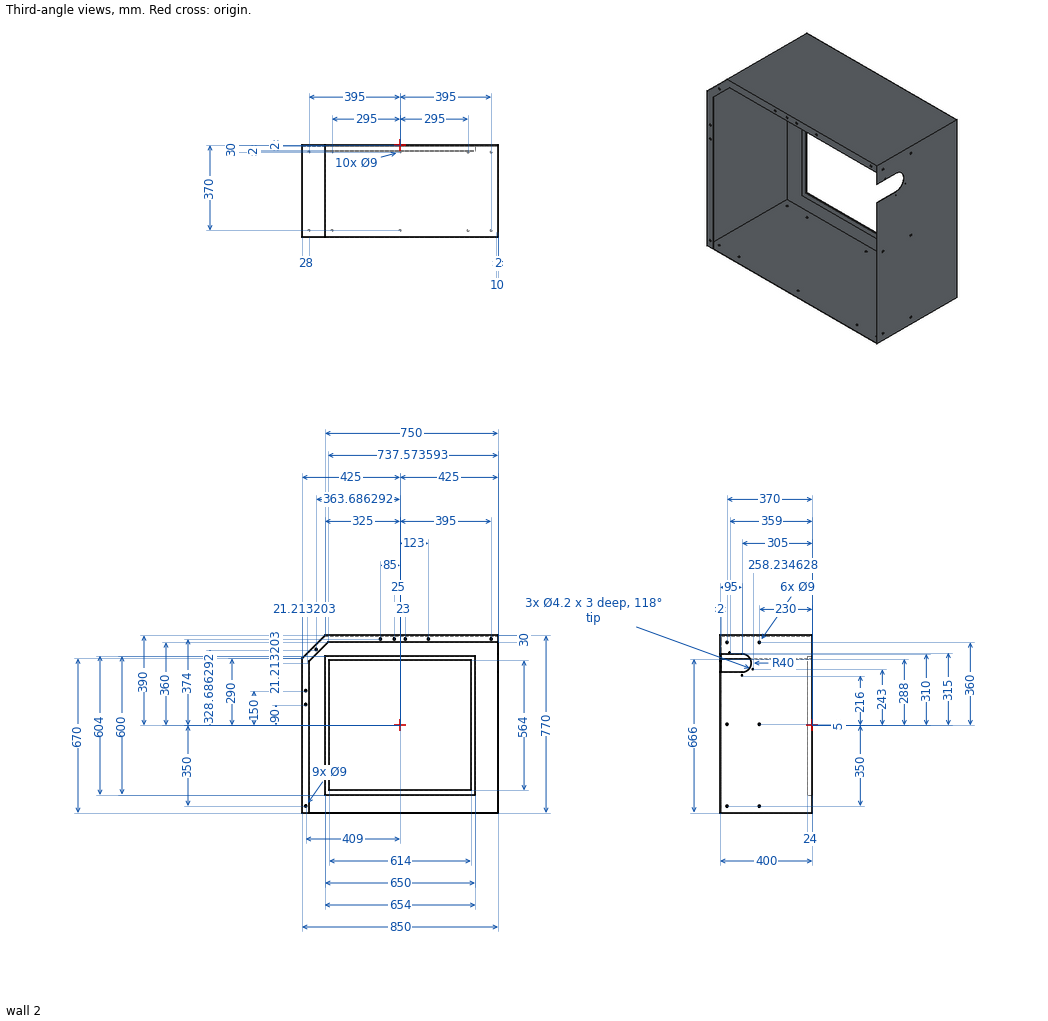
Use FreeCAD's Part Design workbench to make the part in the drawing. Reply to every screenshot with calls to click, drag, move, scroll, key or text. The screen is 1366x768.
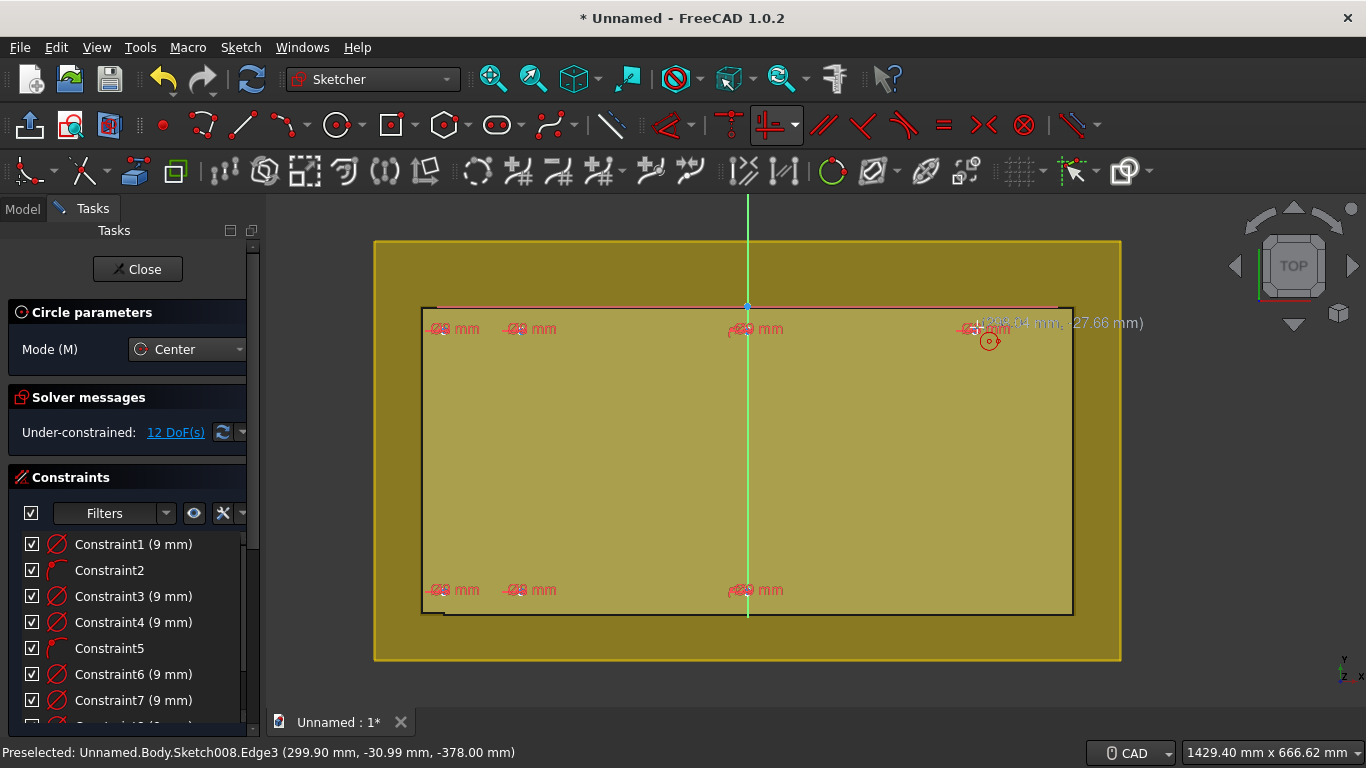
scroll(975, 591, up, 10)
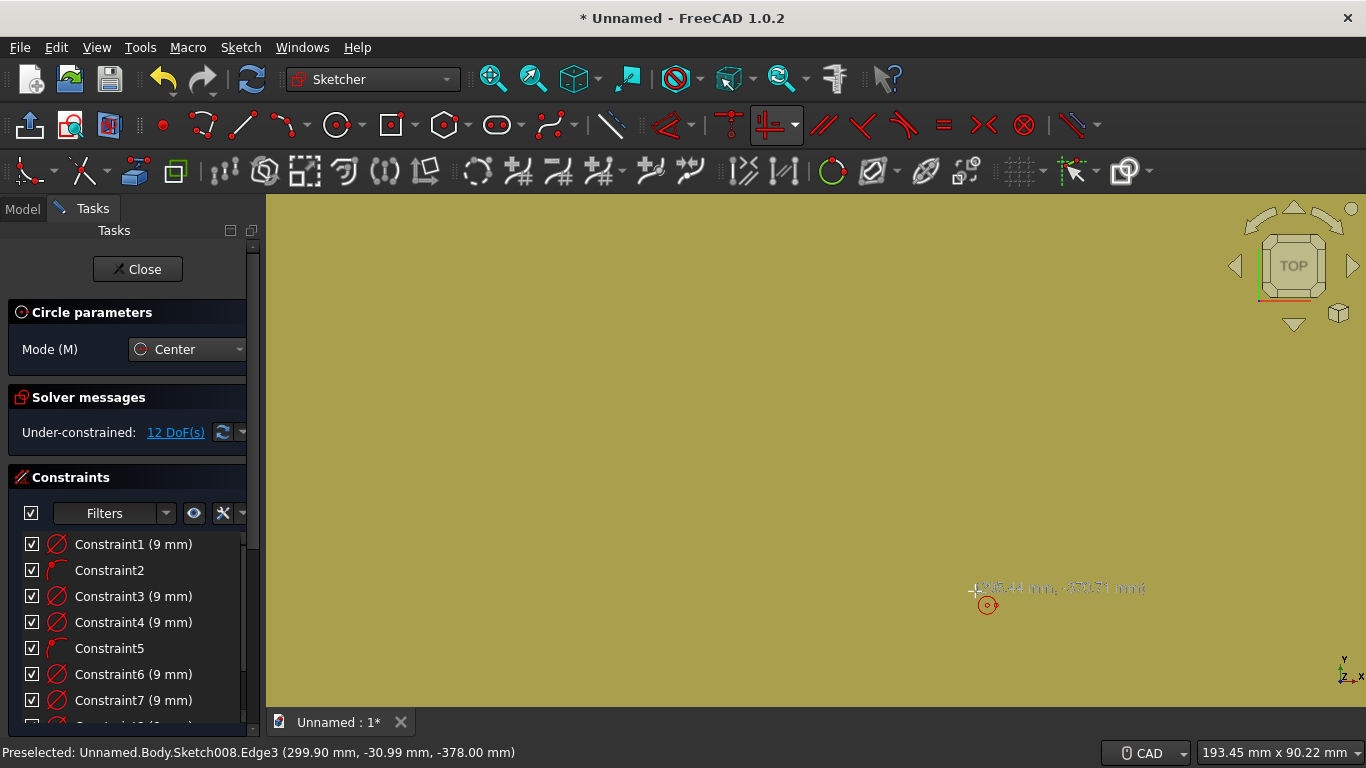
scroll(975, 591, down, 10)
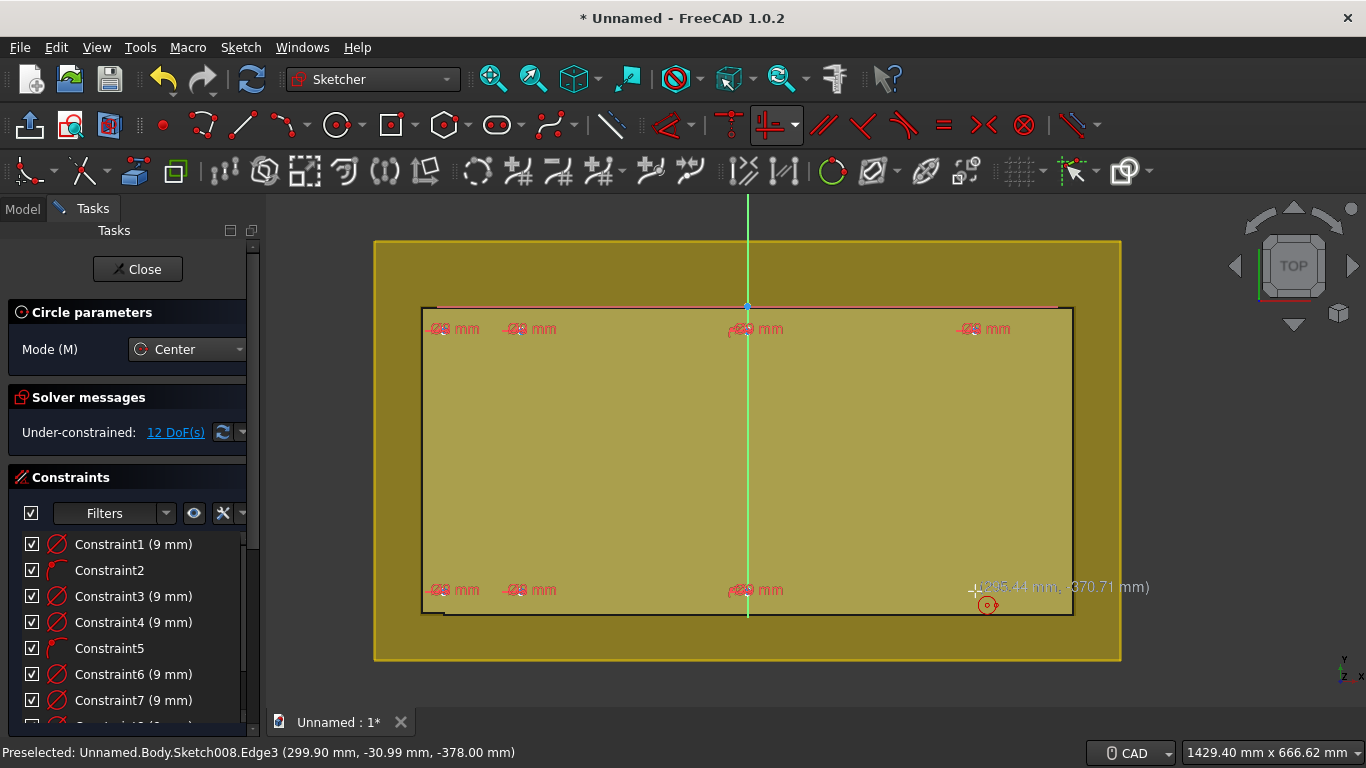
click(975, 591)
move(977, 589)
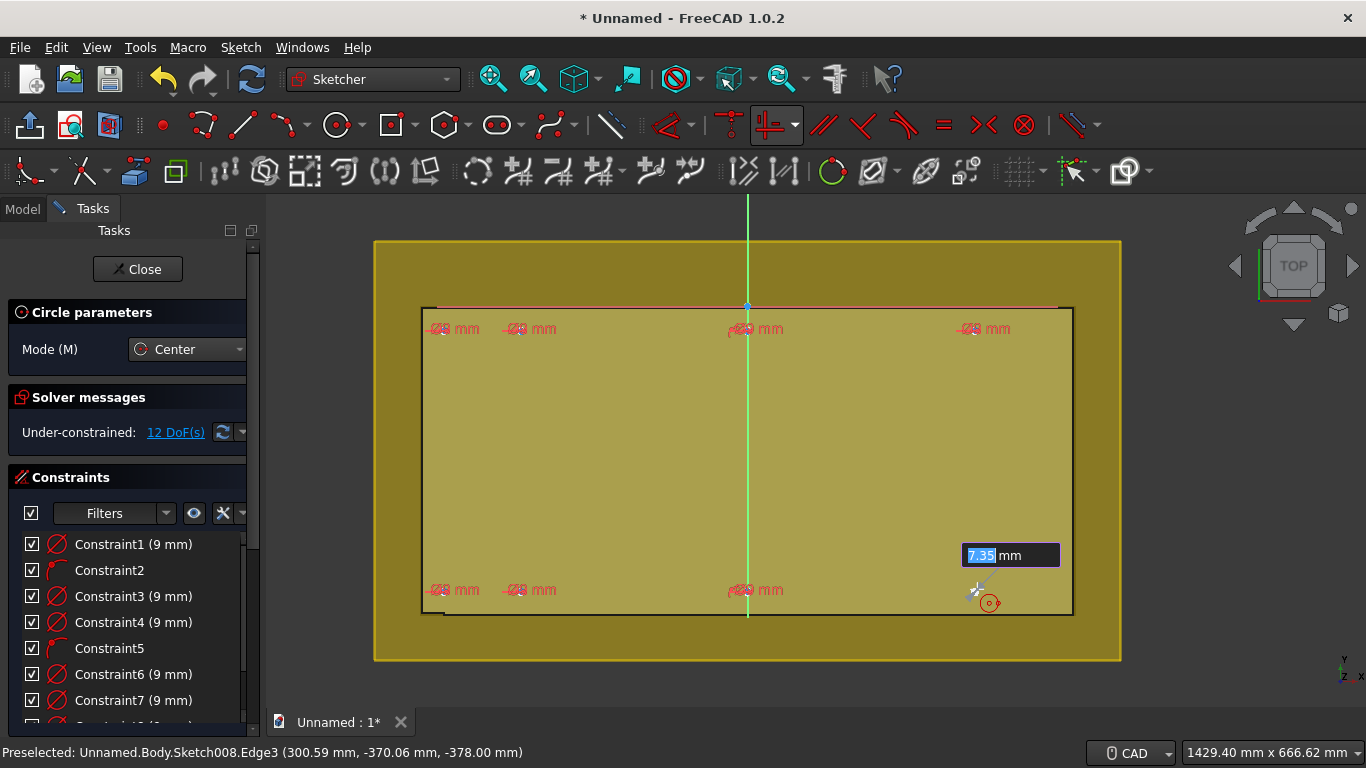
text(9)
key(Return)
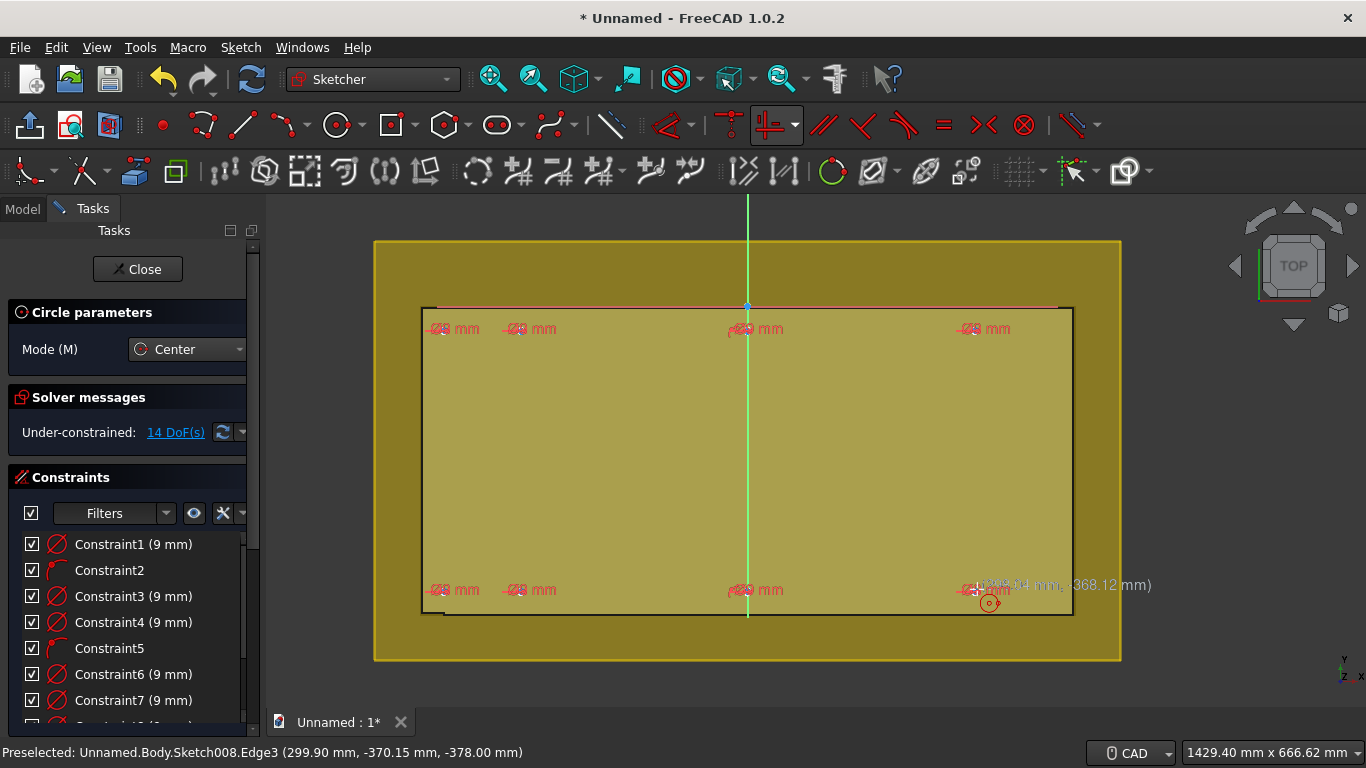
scroll(1052, 591, up, 10)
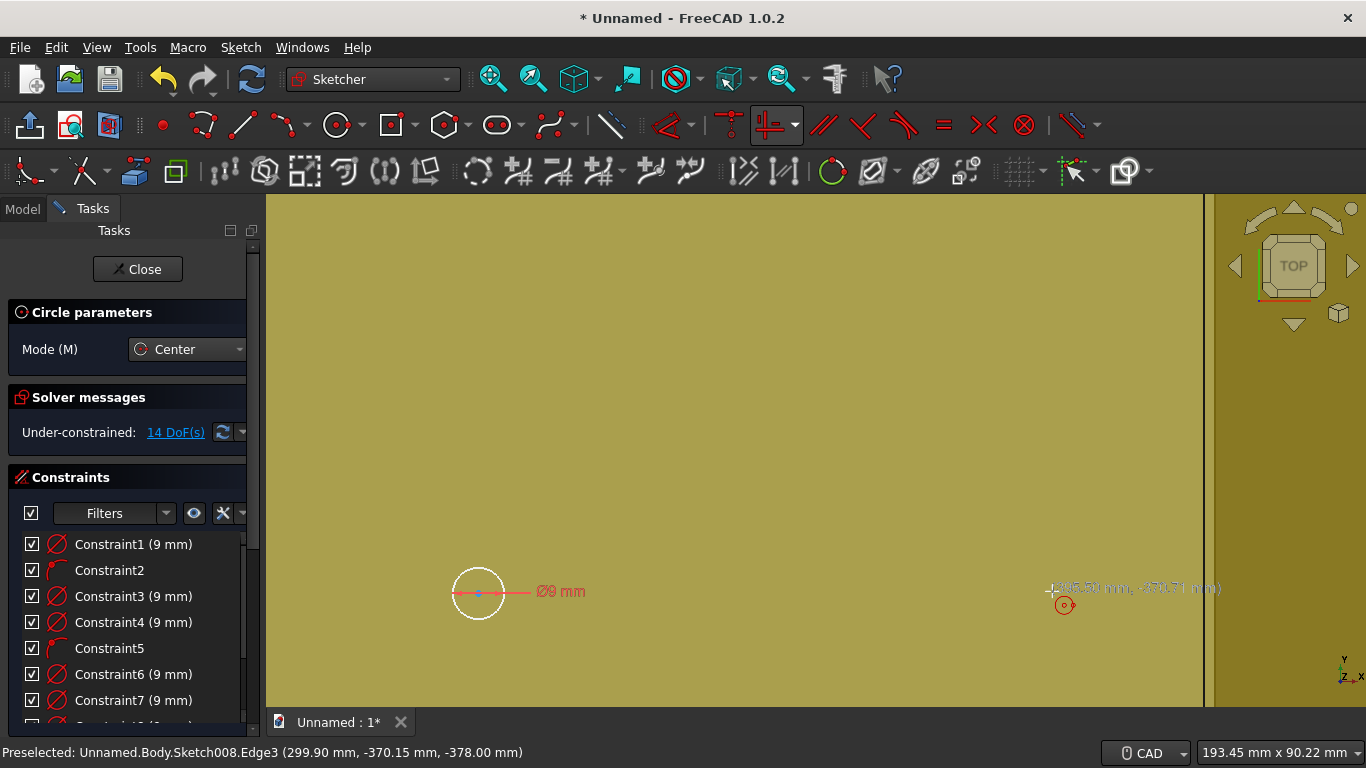
scroll(1053, 591, down, 10)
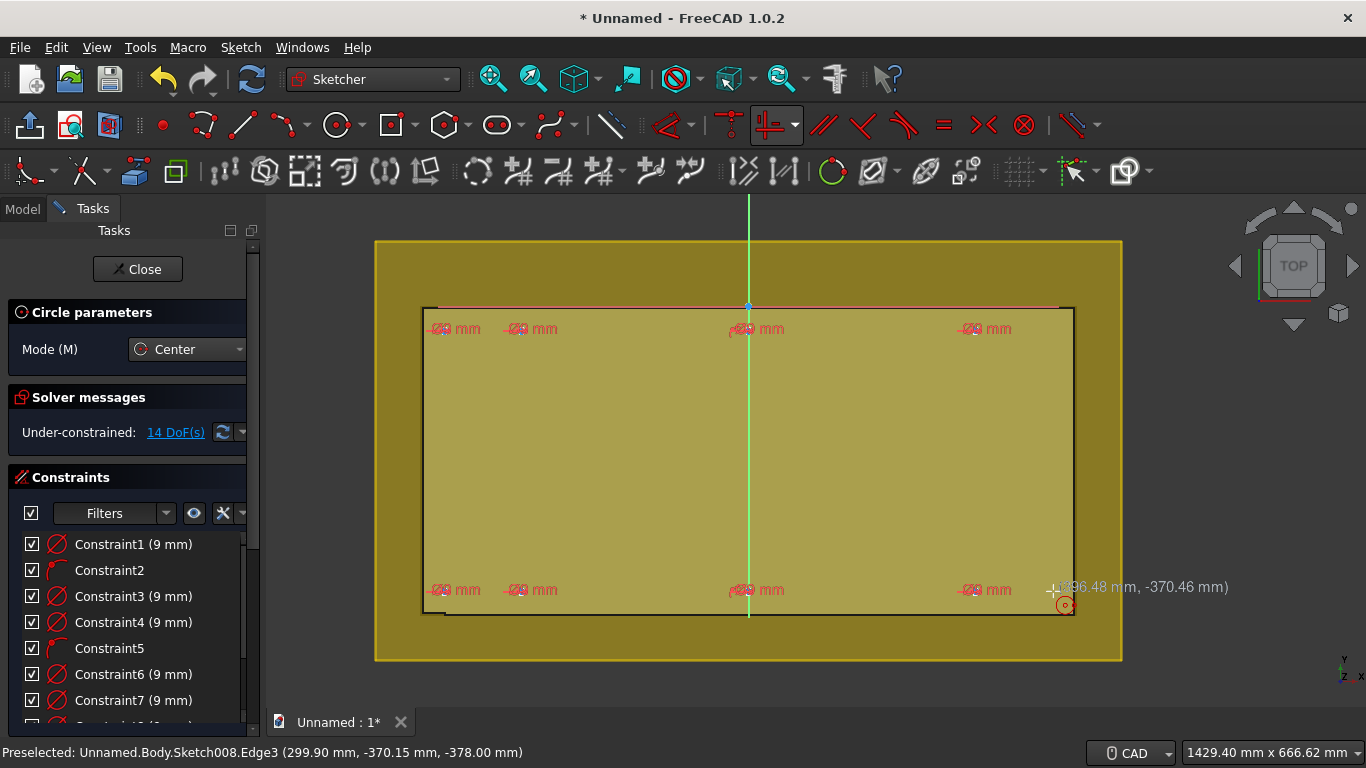
click(1052, 591)
move(1055, 589)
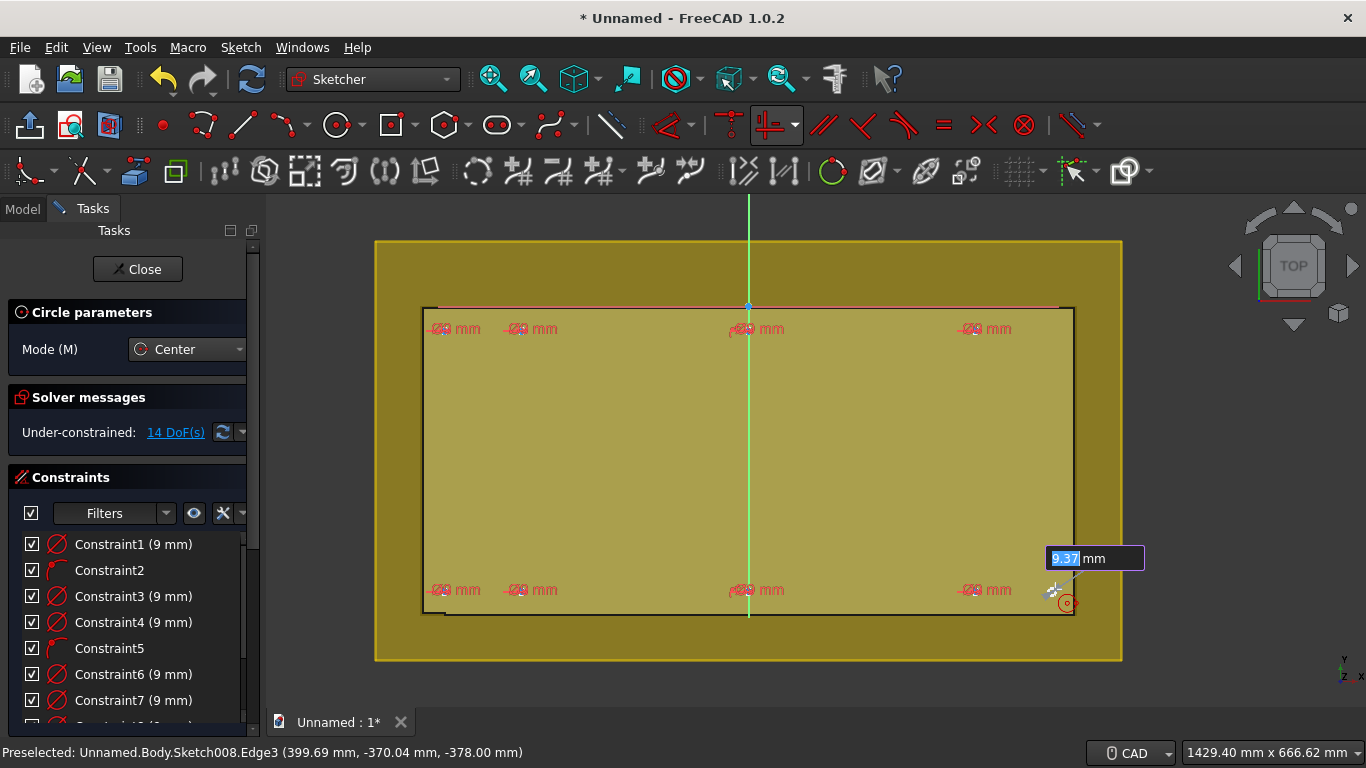
text(9)
key(Return)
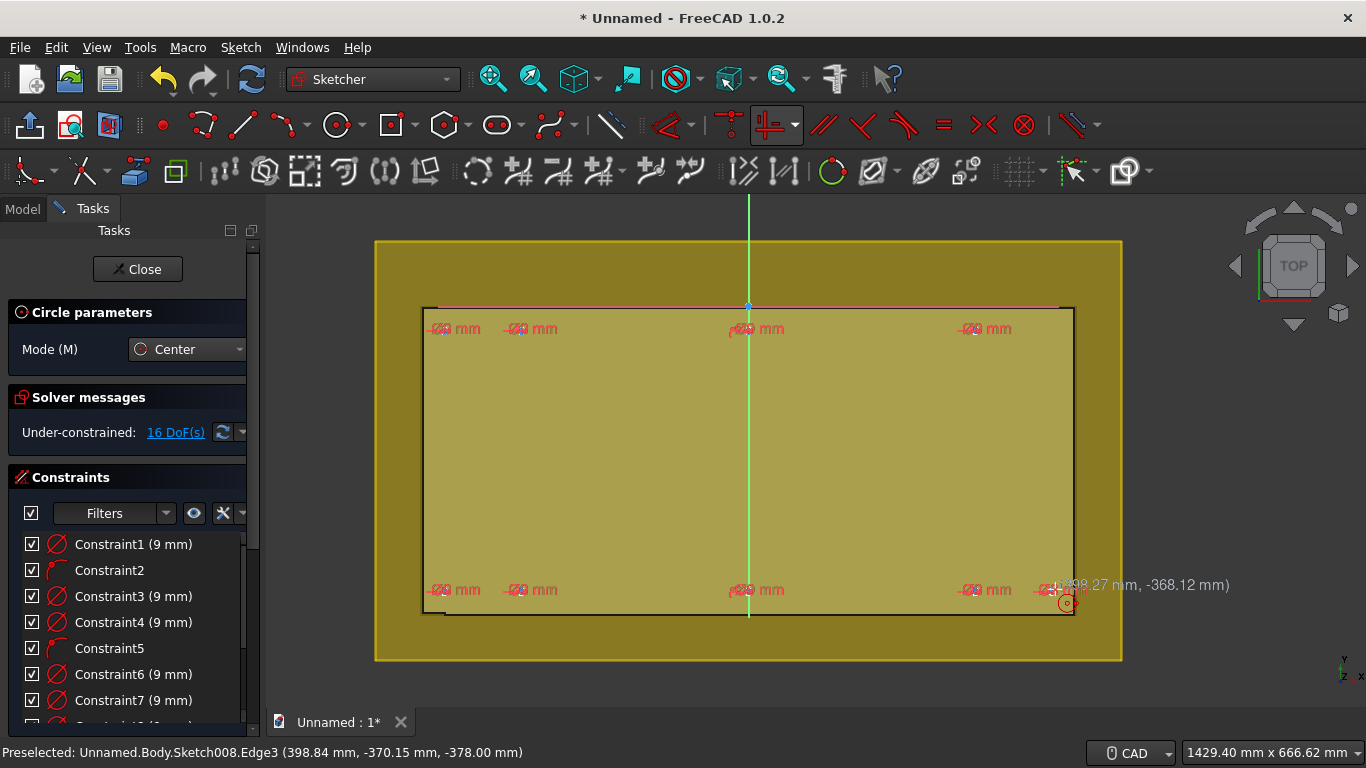
scroll(1052, 330, up, 10)